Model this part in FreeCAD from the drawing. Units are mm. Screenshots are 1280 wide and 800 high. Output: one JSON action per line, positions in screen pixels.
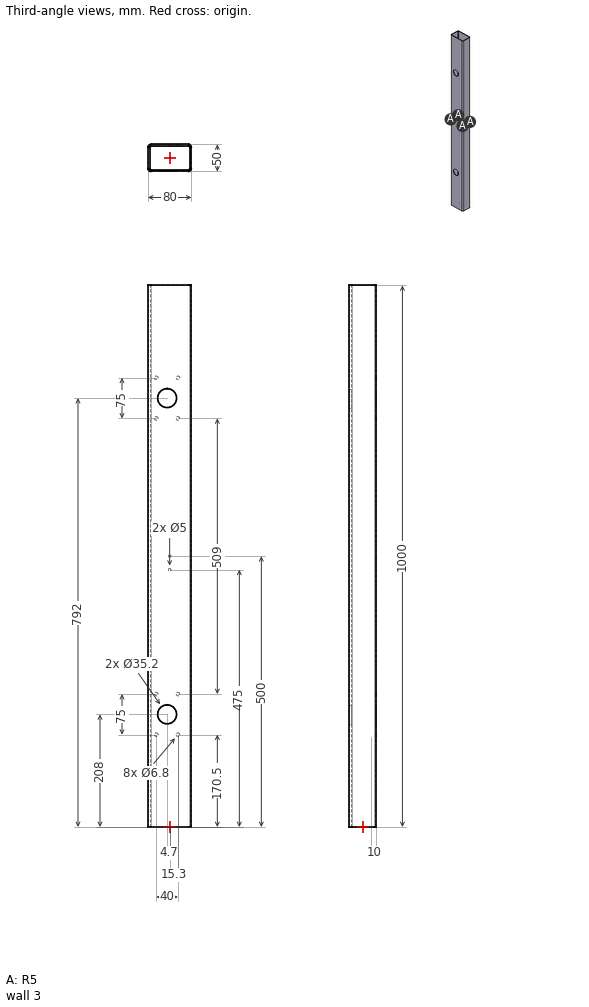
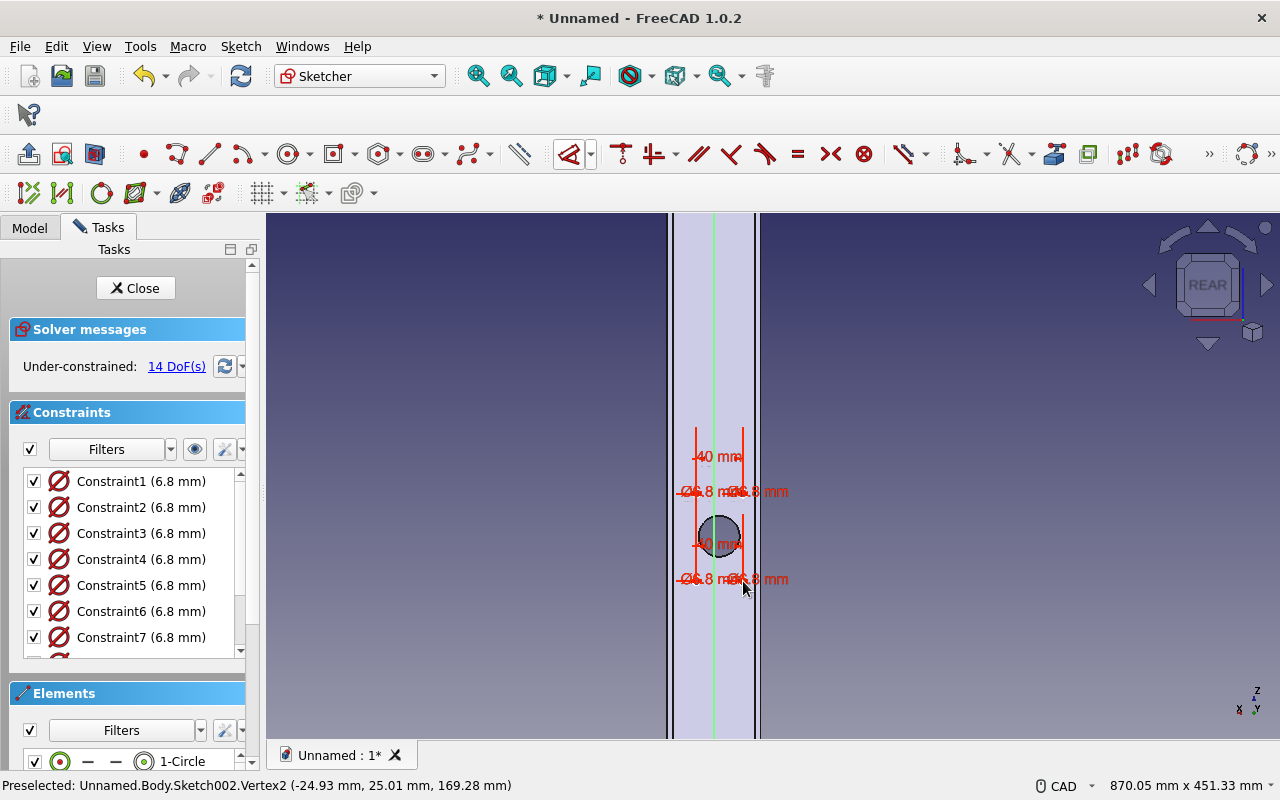
{"action": "left_click", "coordinate": [743, 494]}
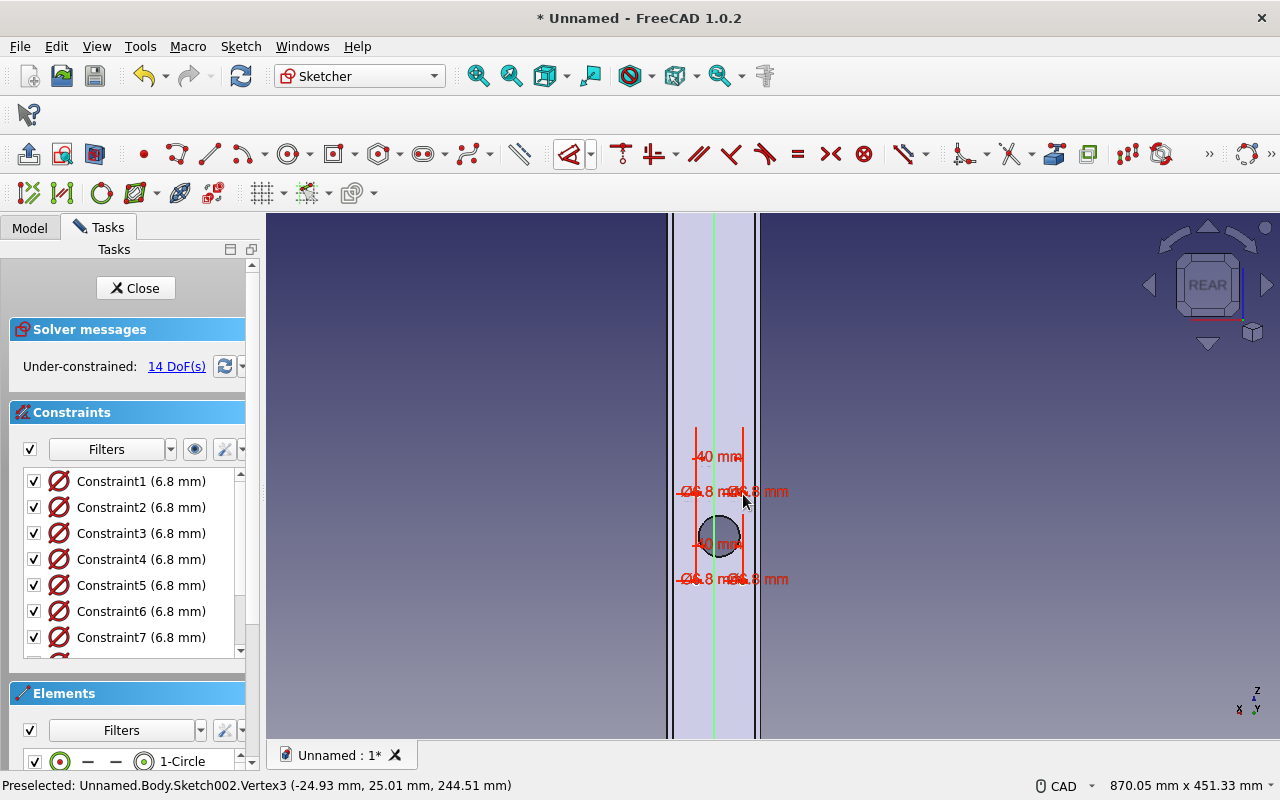
{"action": "left_click", "coordinate": [590, 154]}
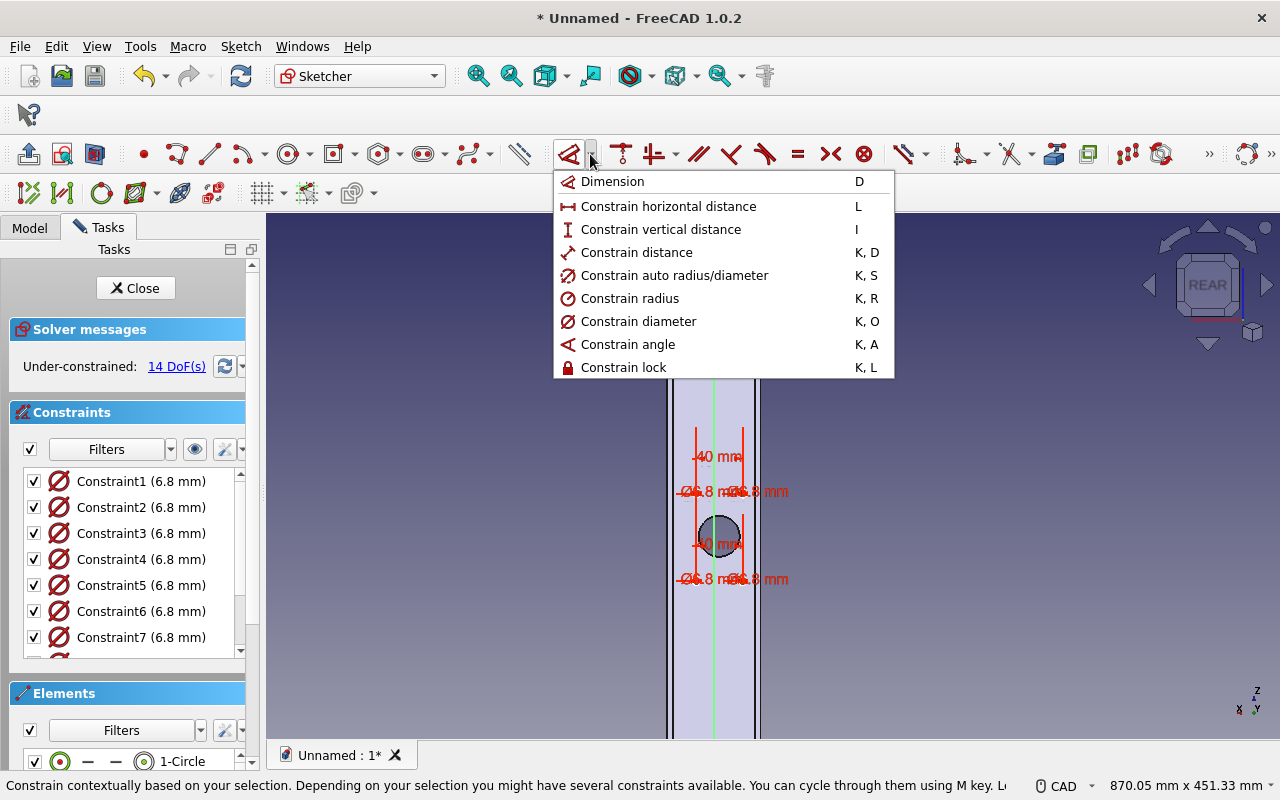
{"action": "left_click", "coordinate": [724, 230]}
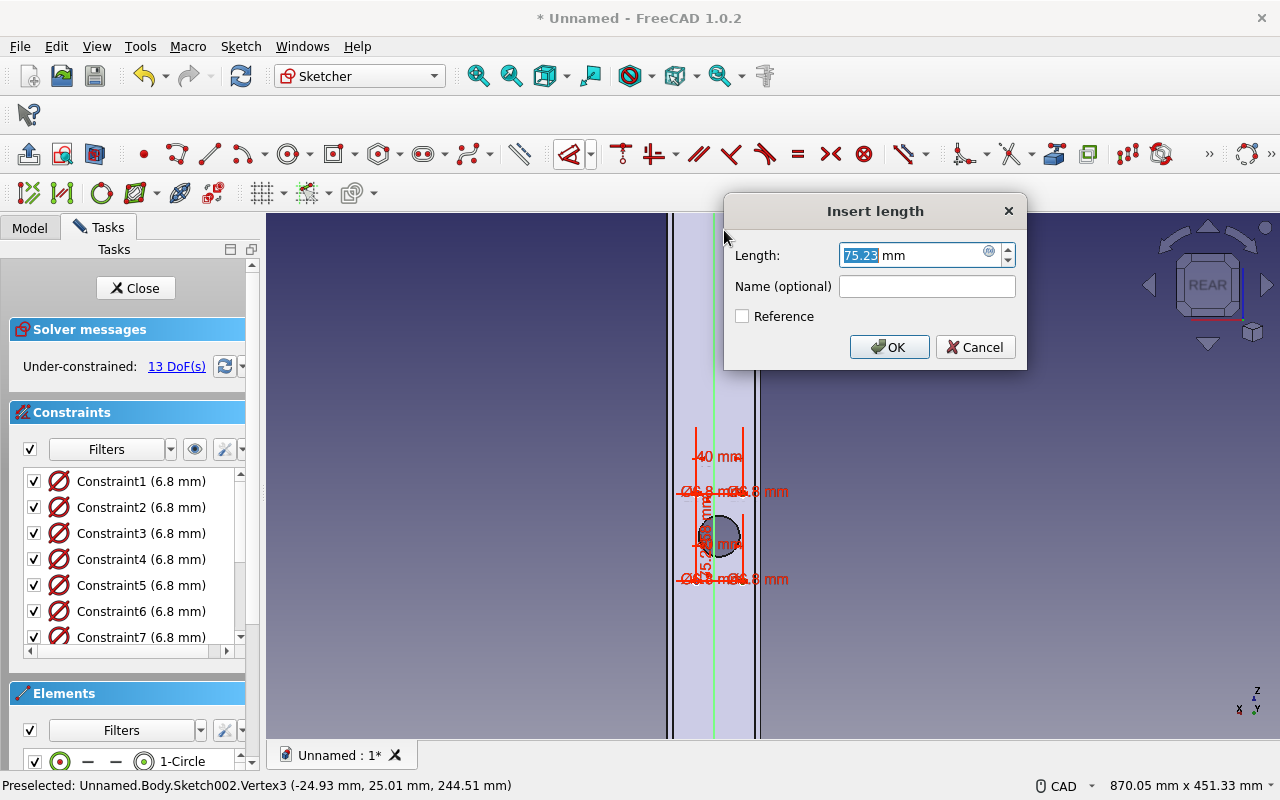
{"action": "type", "text": "75"}
{"action": "key", "text": "Return"}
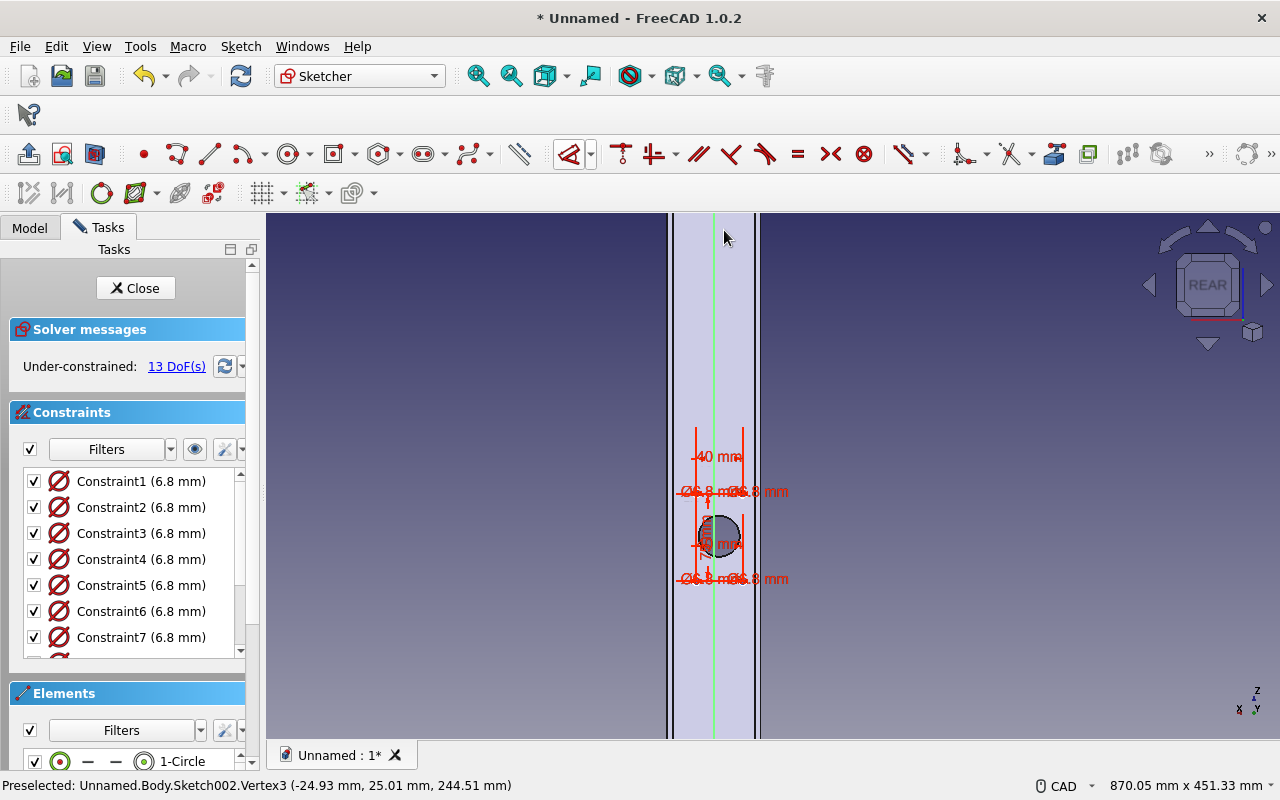
{"action": "left_click", "coordinate": [696, 581]}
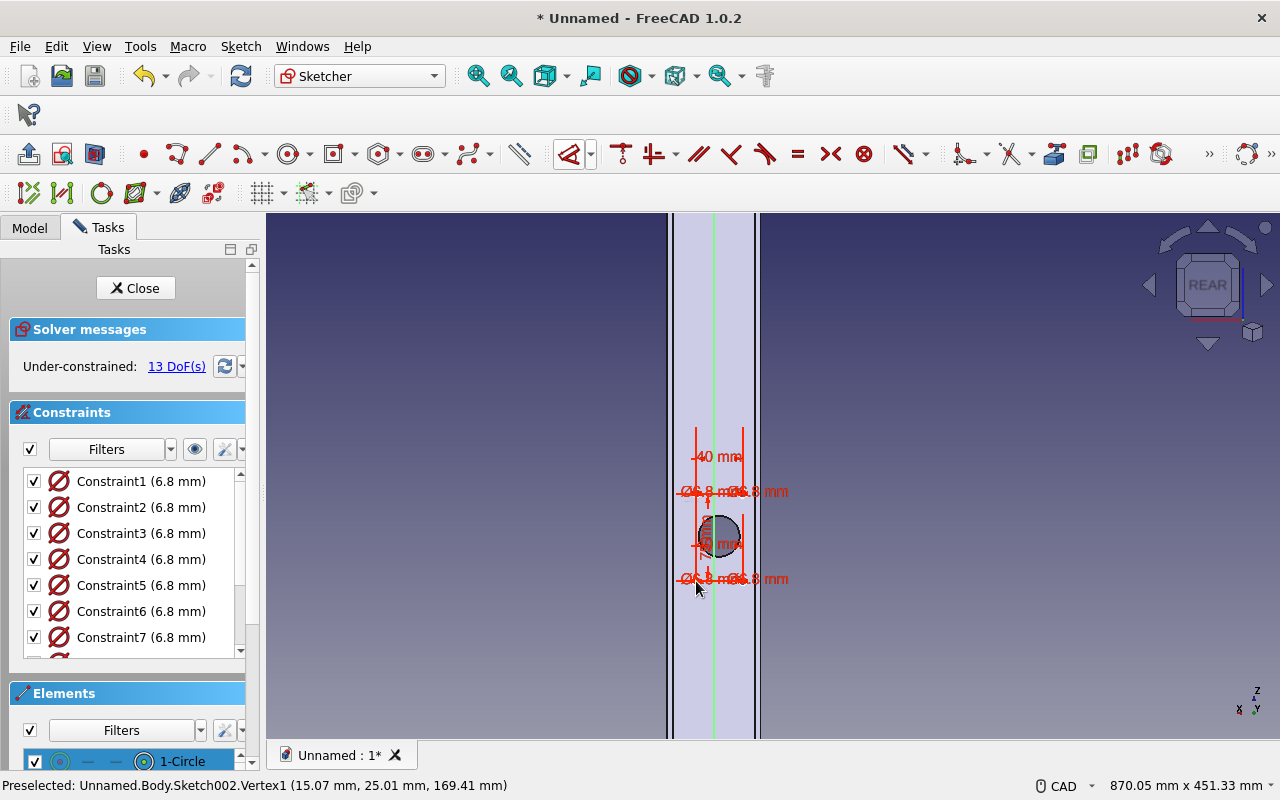
{"action": "left_click", "coordinate": [743, 494]}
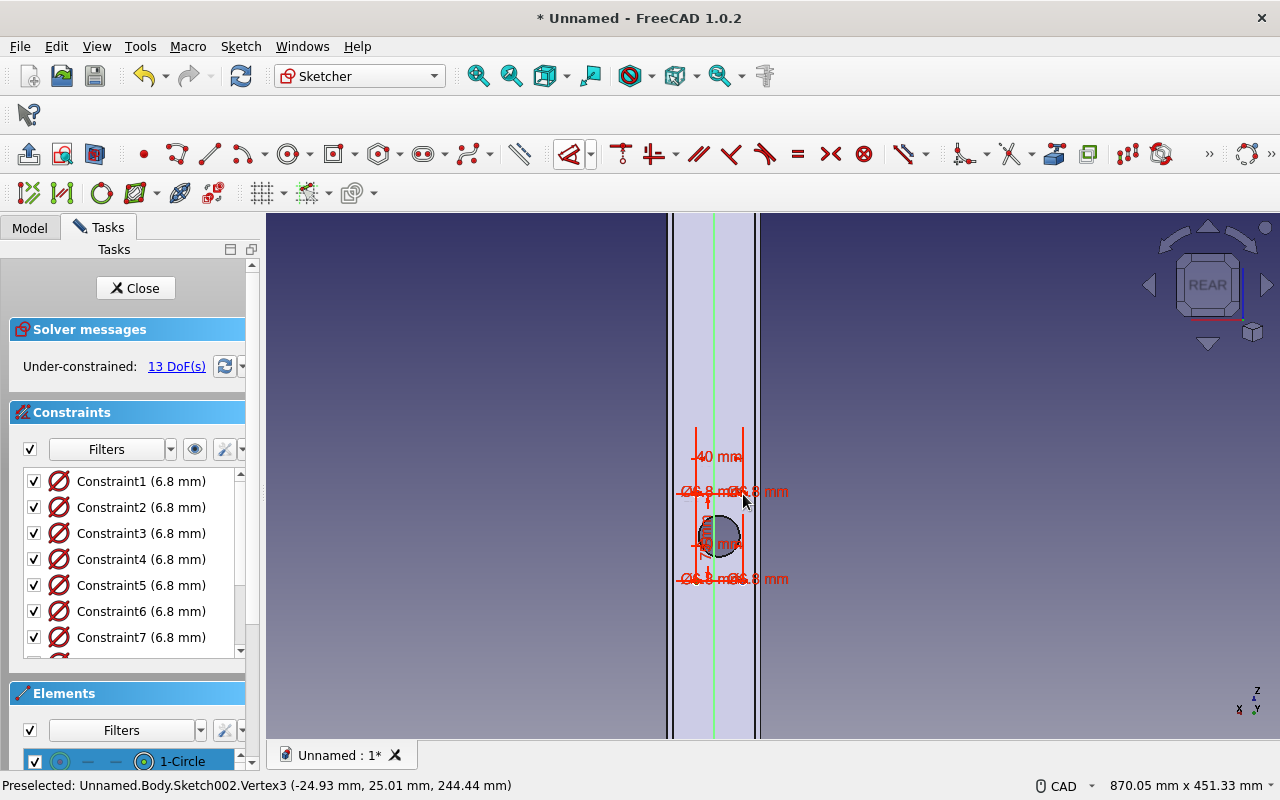
{"action": "left_click", "coordinate": [590, 154]}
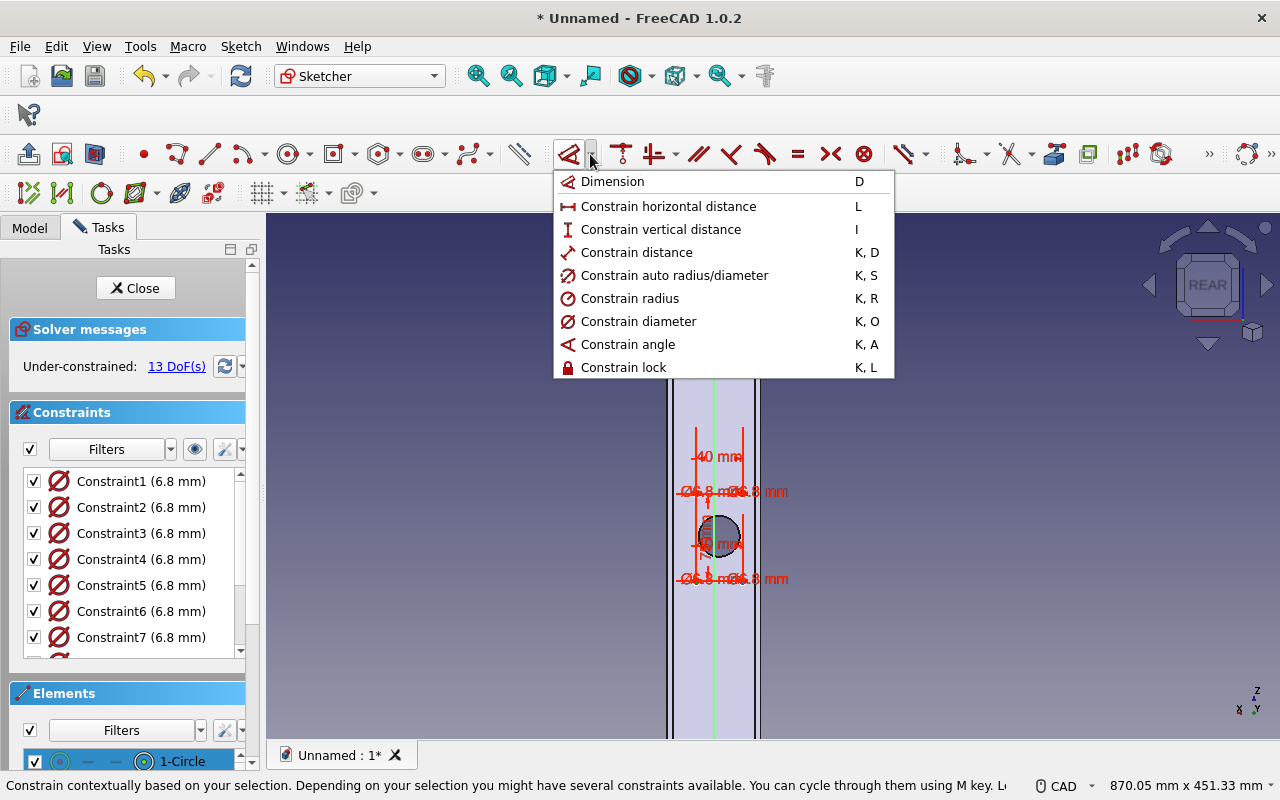
{"action": "left_click", "coordinate": [724, 230]}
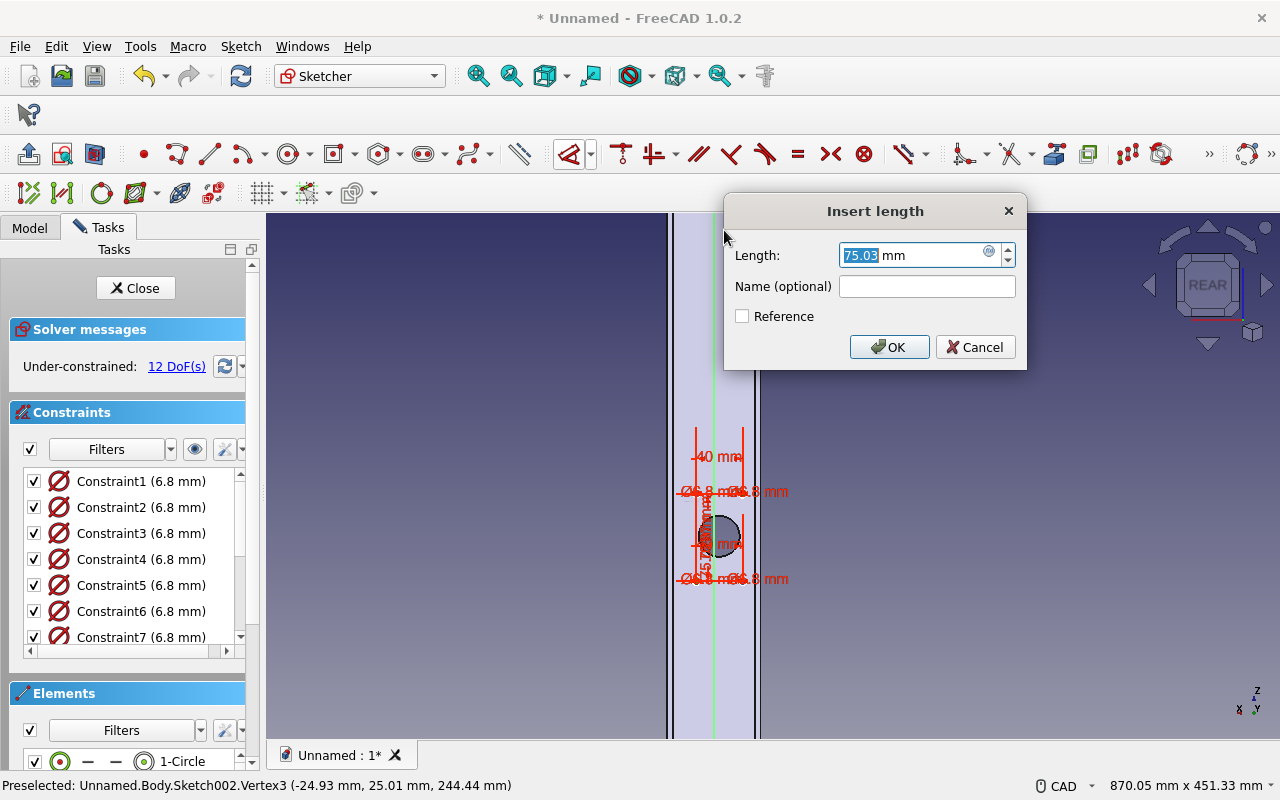
{"action": "type", "text": "75"}
{"action": "key", "text": "Return"}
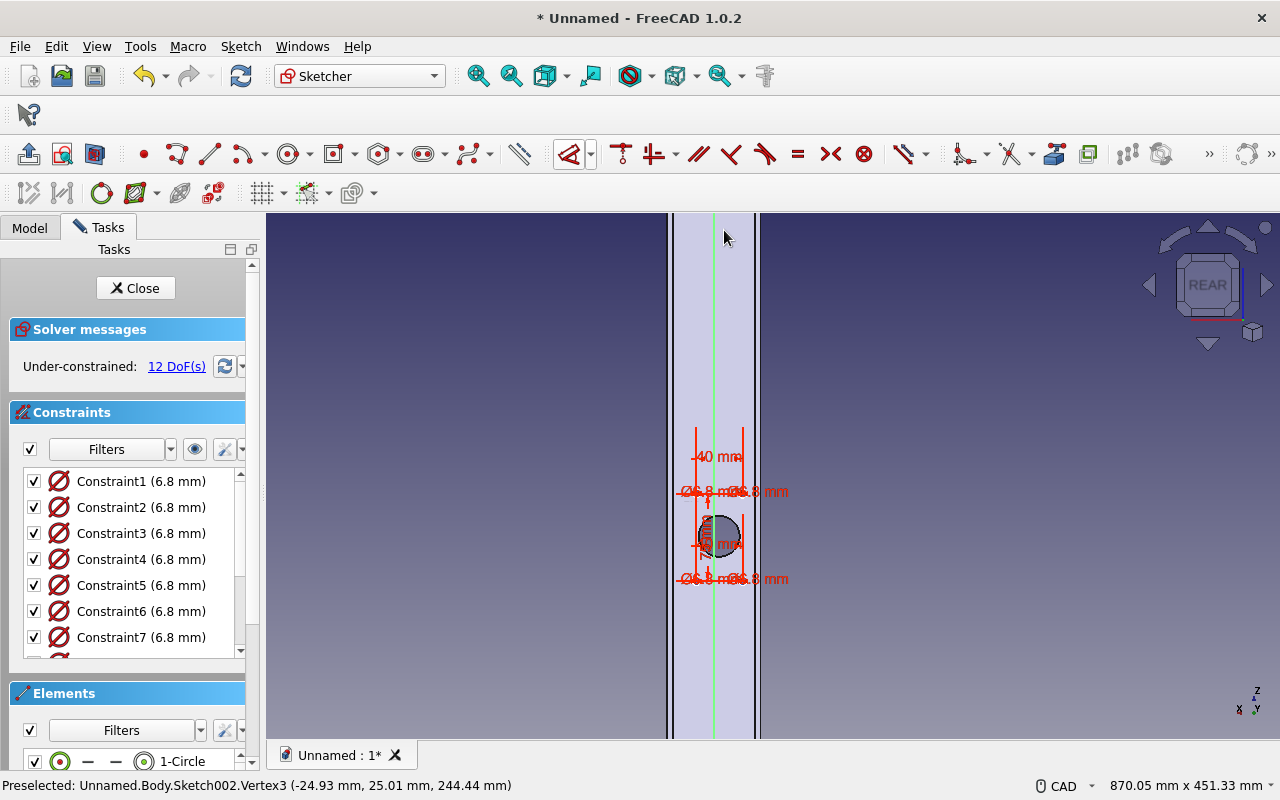
{"action": "left_click", "coordinate": [743, 494]}